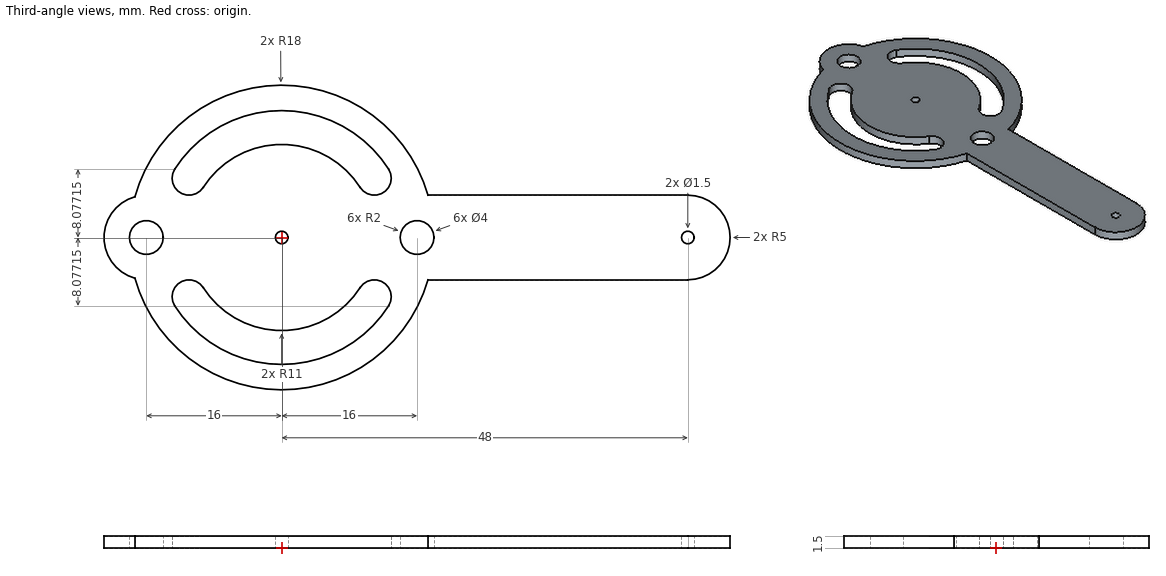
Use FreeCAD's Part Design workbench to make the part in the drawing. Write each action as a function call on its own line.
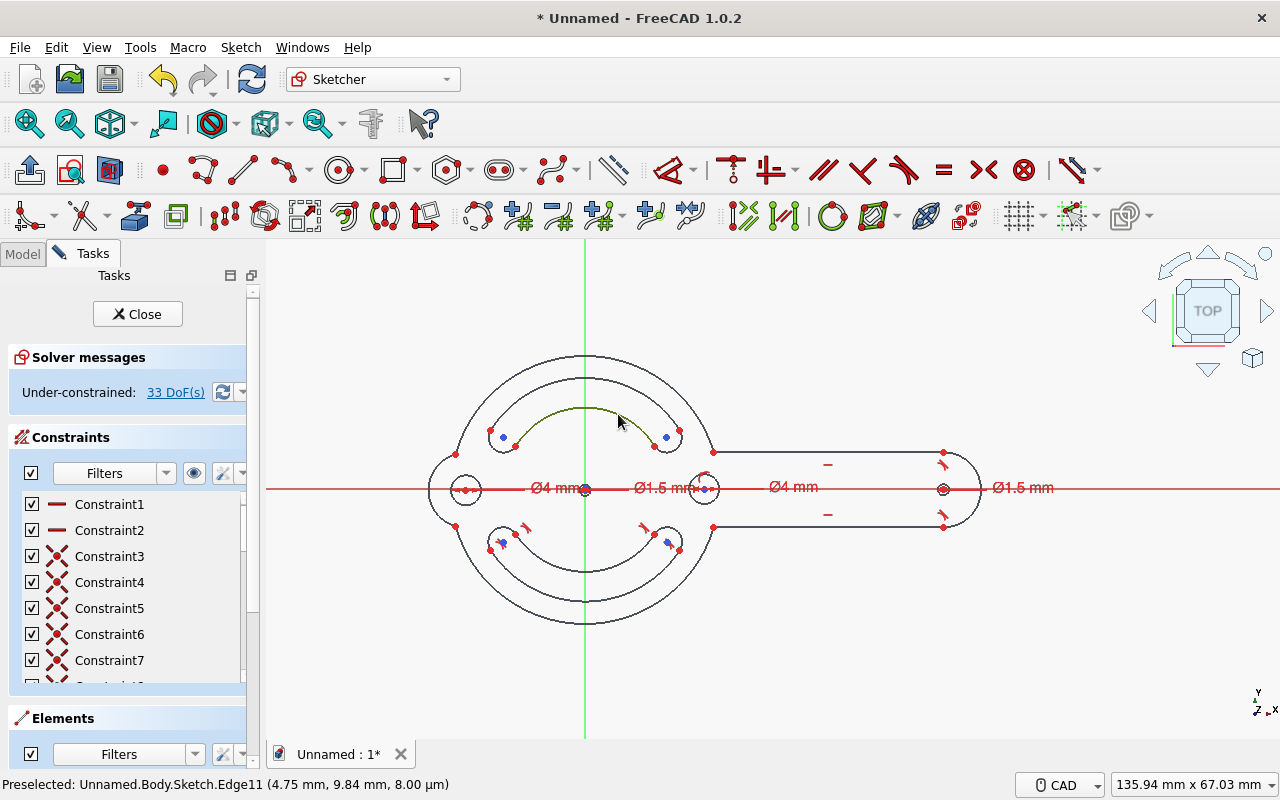
click(490, 443)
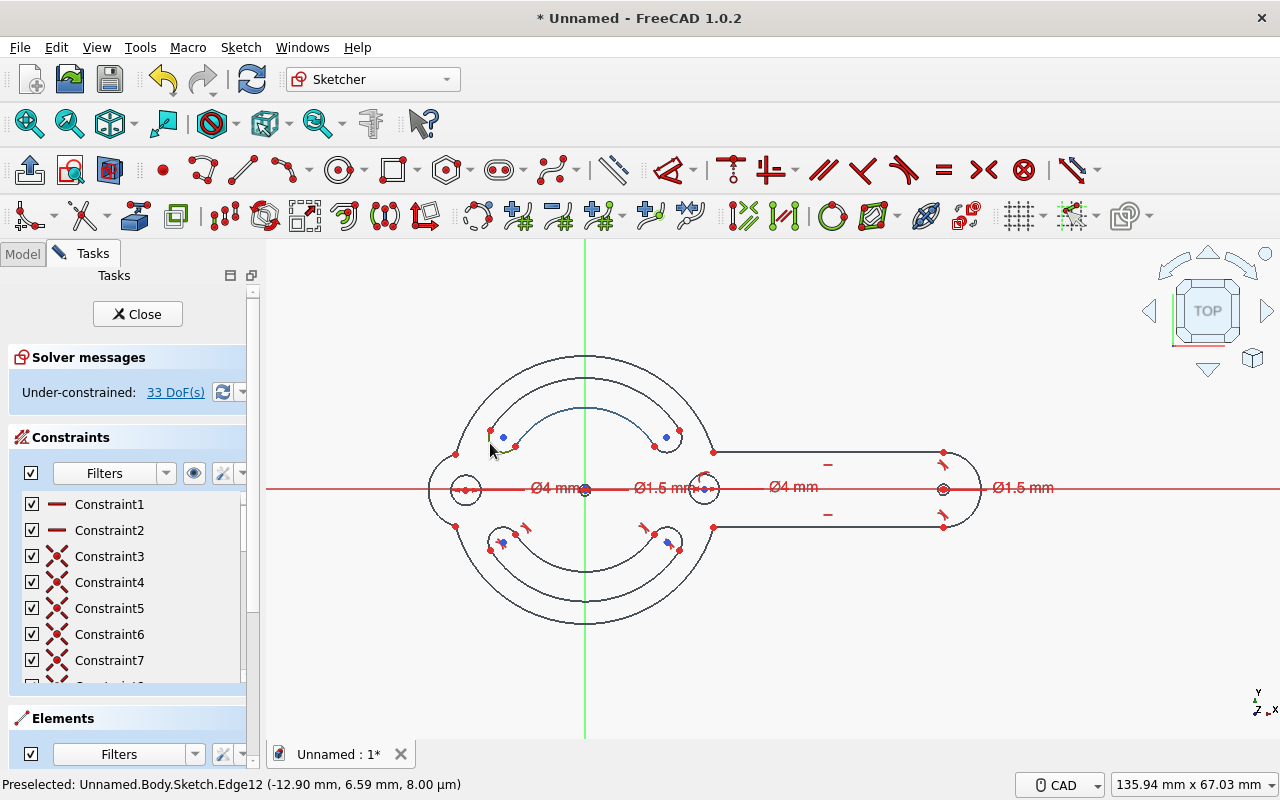
click(904, 170)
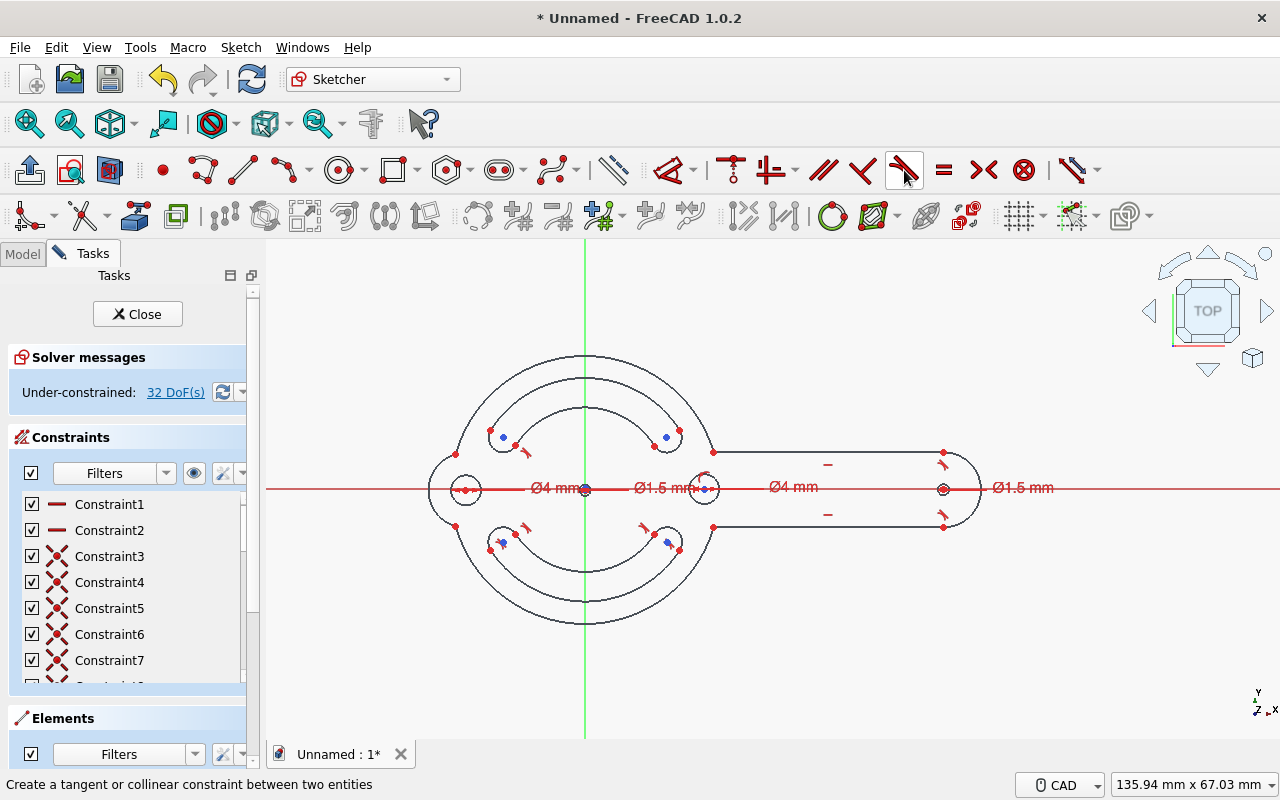
click(618, 414)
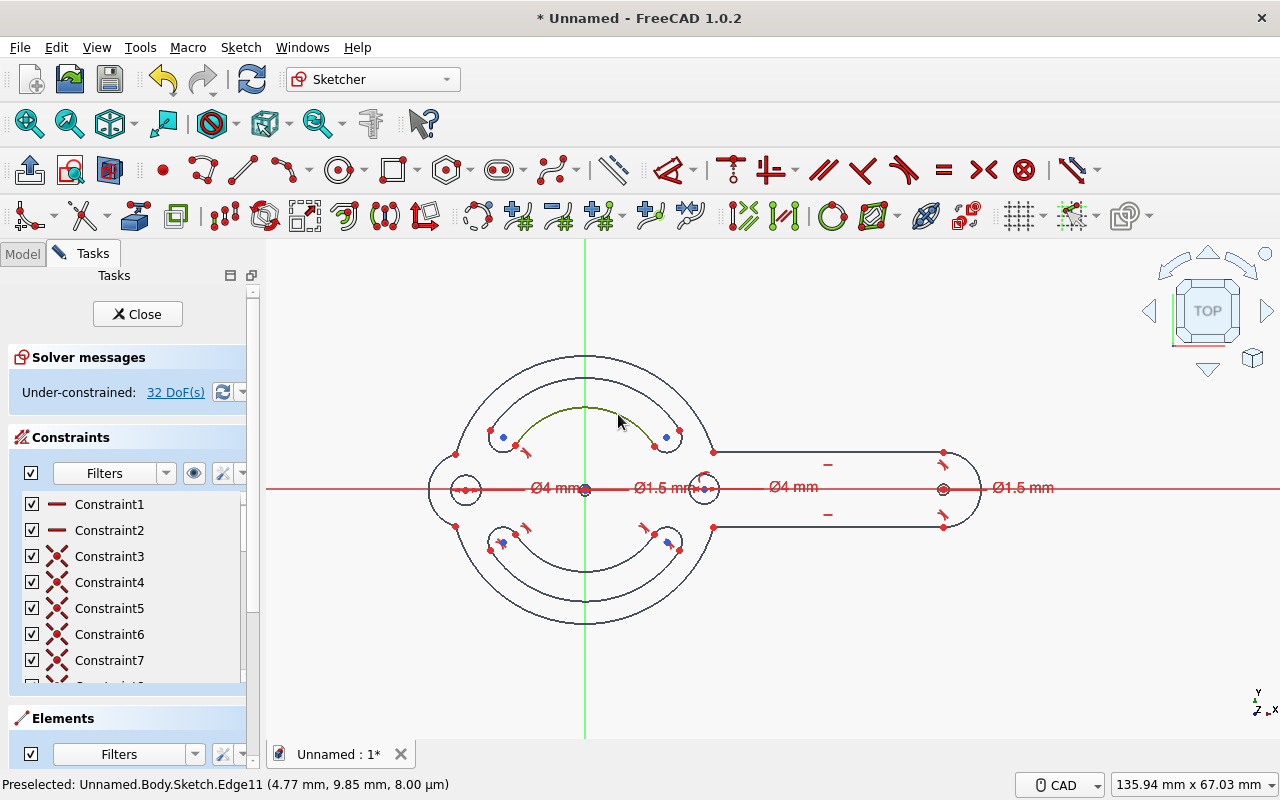
click(666, 453)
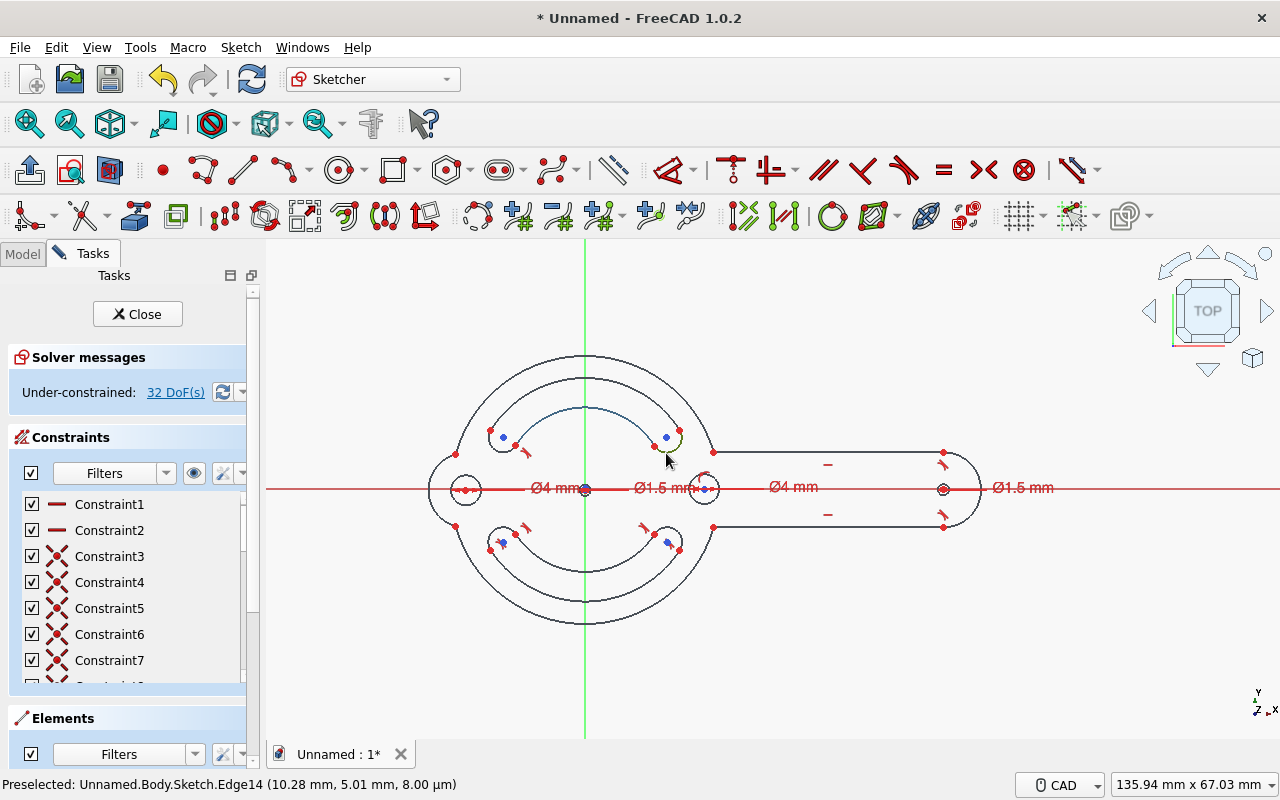
click(904, 170)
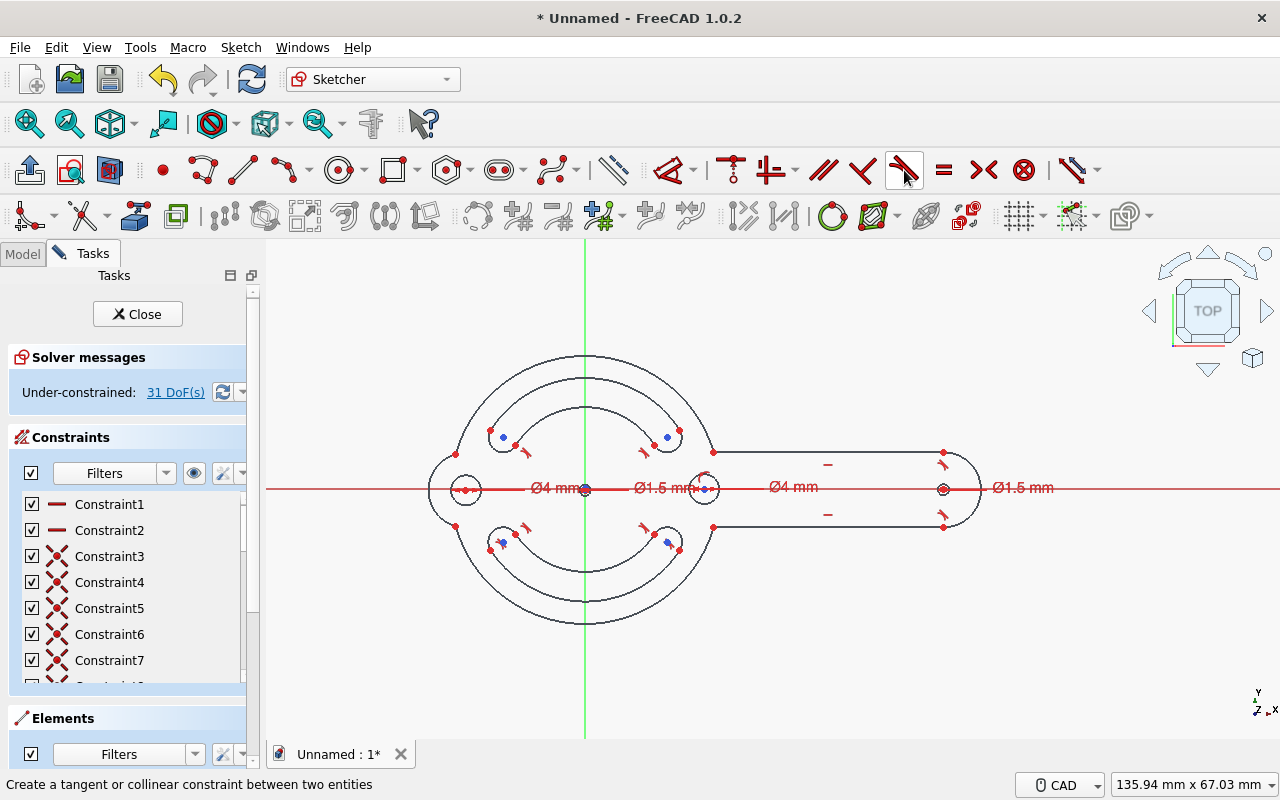
click(490, 443)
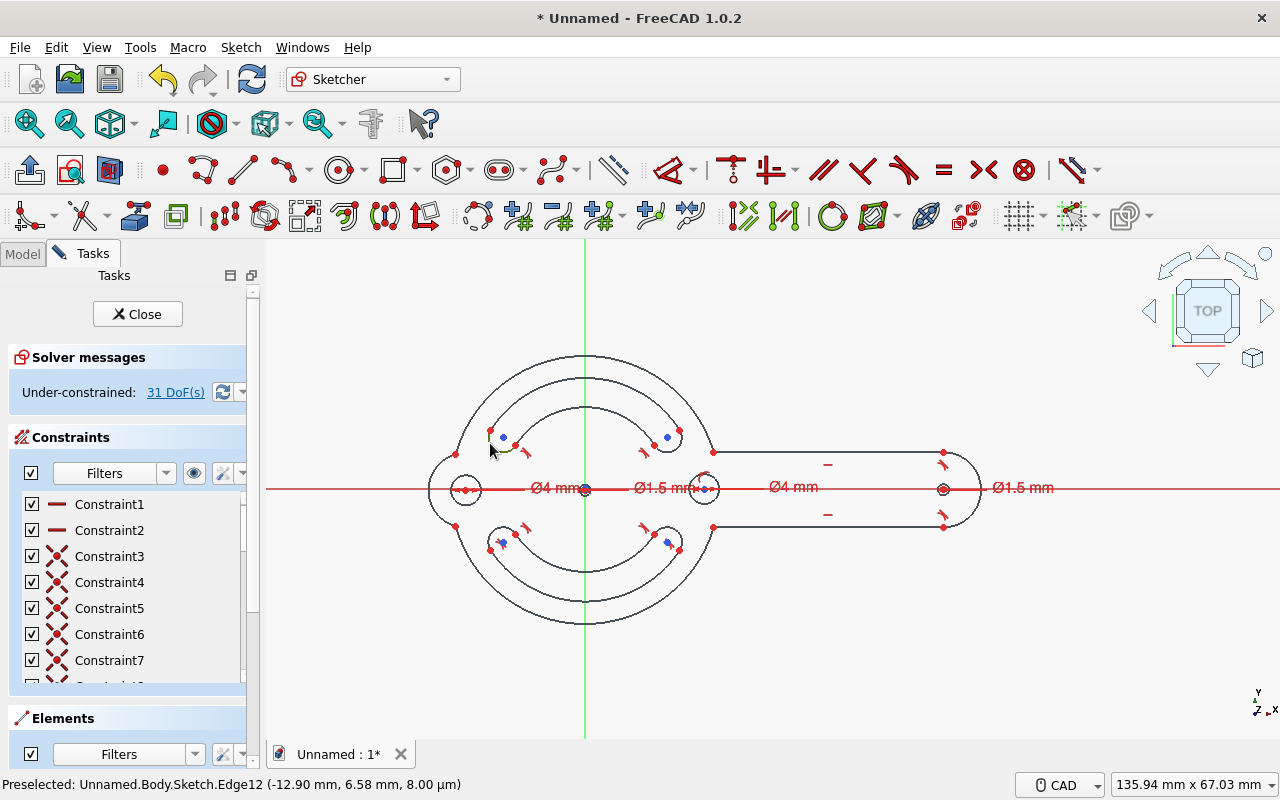
click(629, 387)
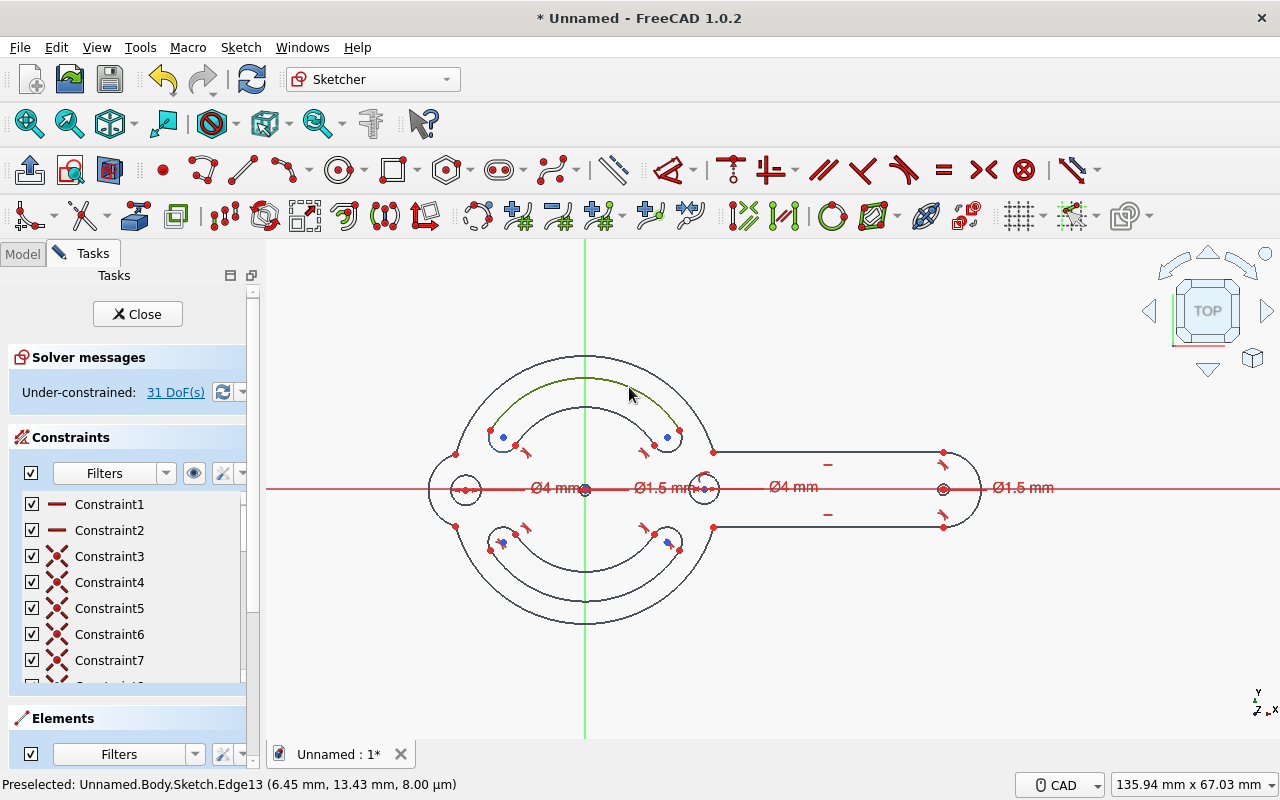
click(904, 170)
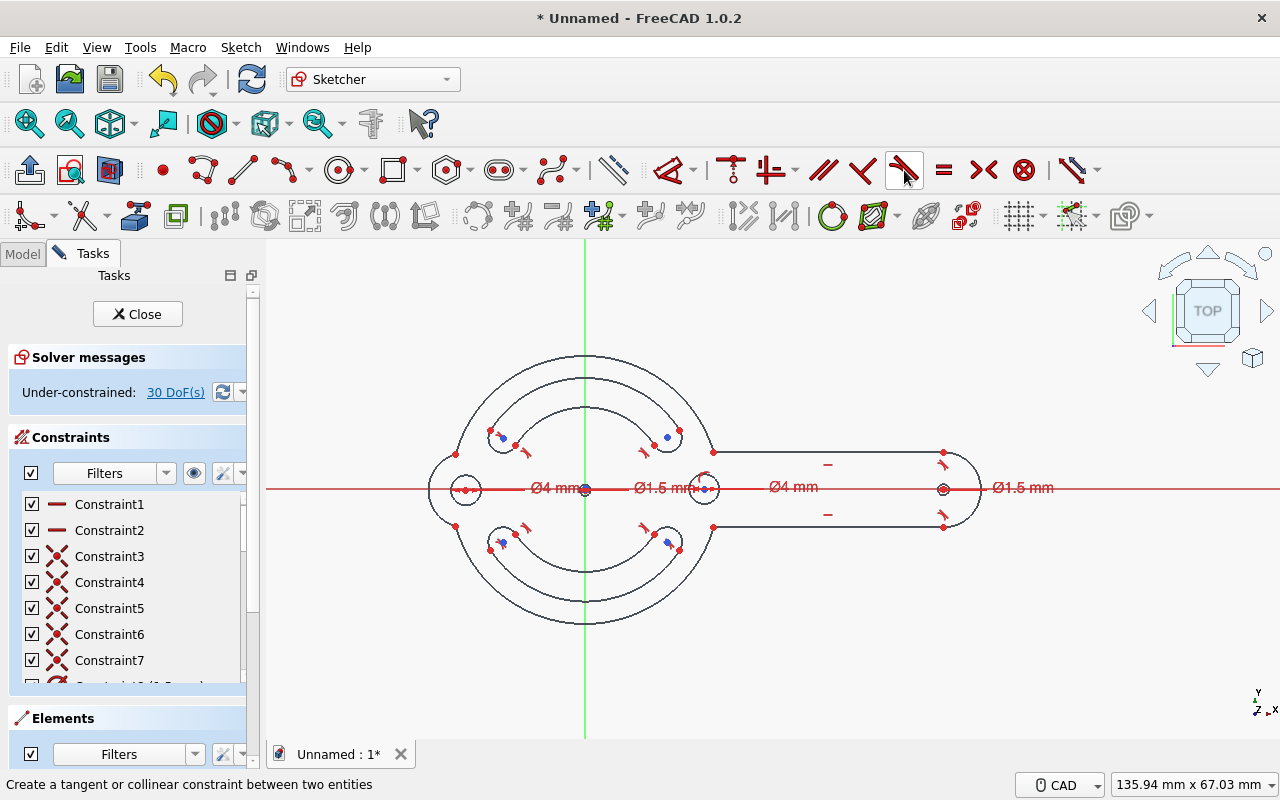
click(629, 387)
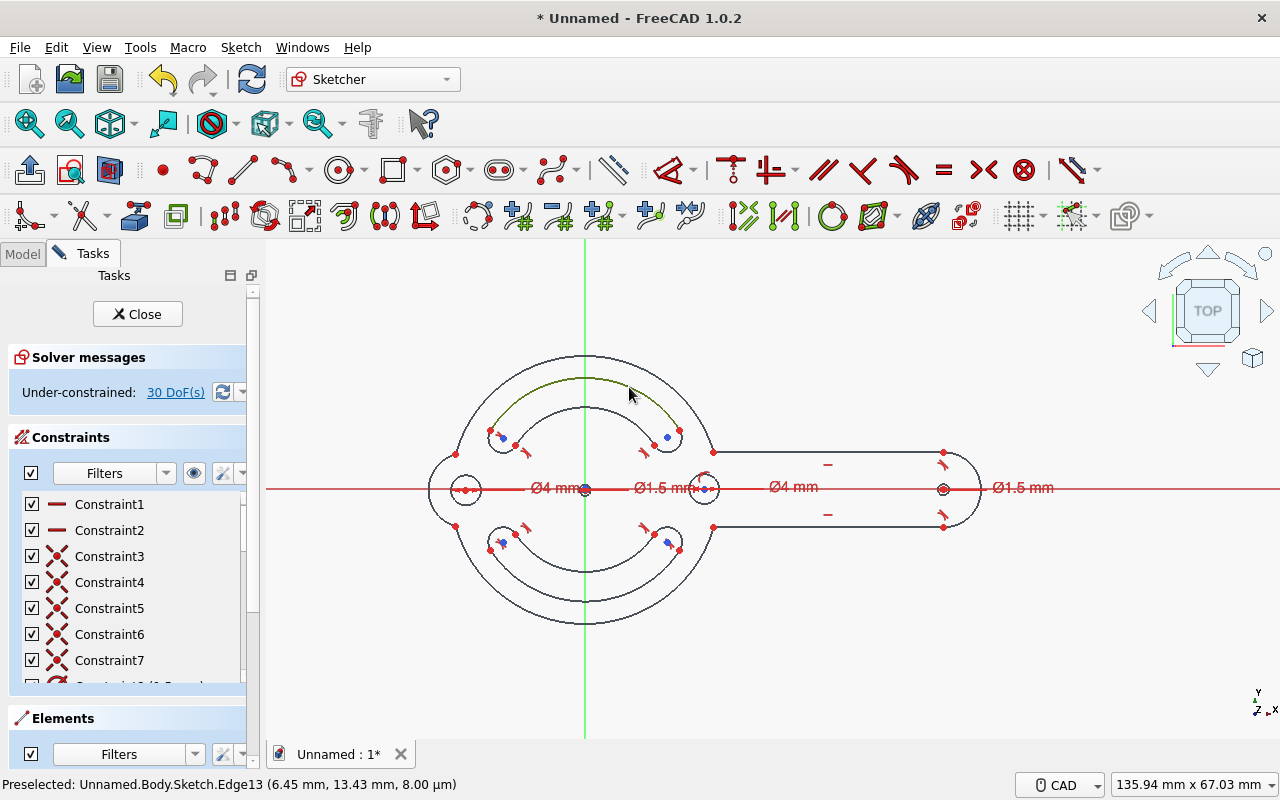
click(666, 452)